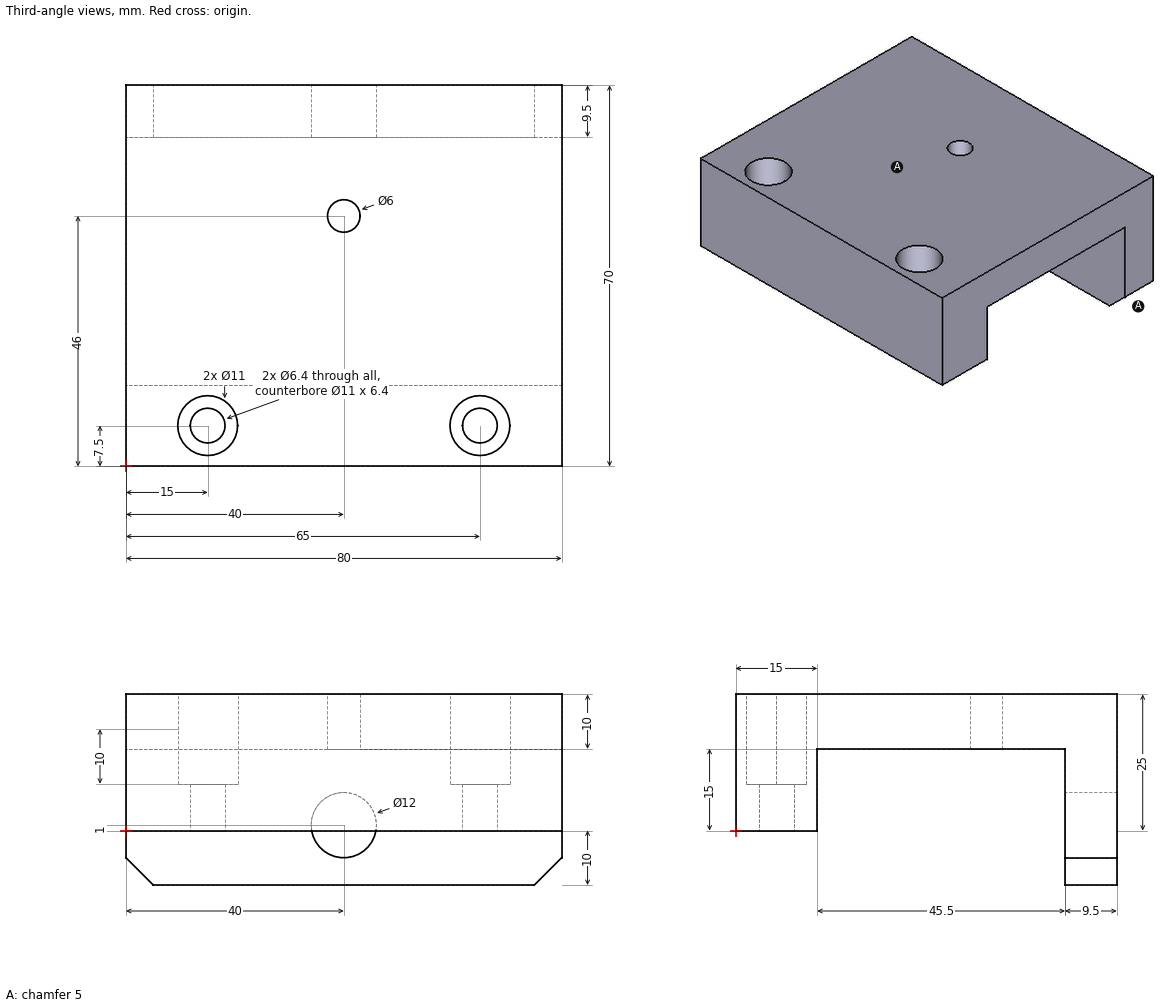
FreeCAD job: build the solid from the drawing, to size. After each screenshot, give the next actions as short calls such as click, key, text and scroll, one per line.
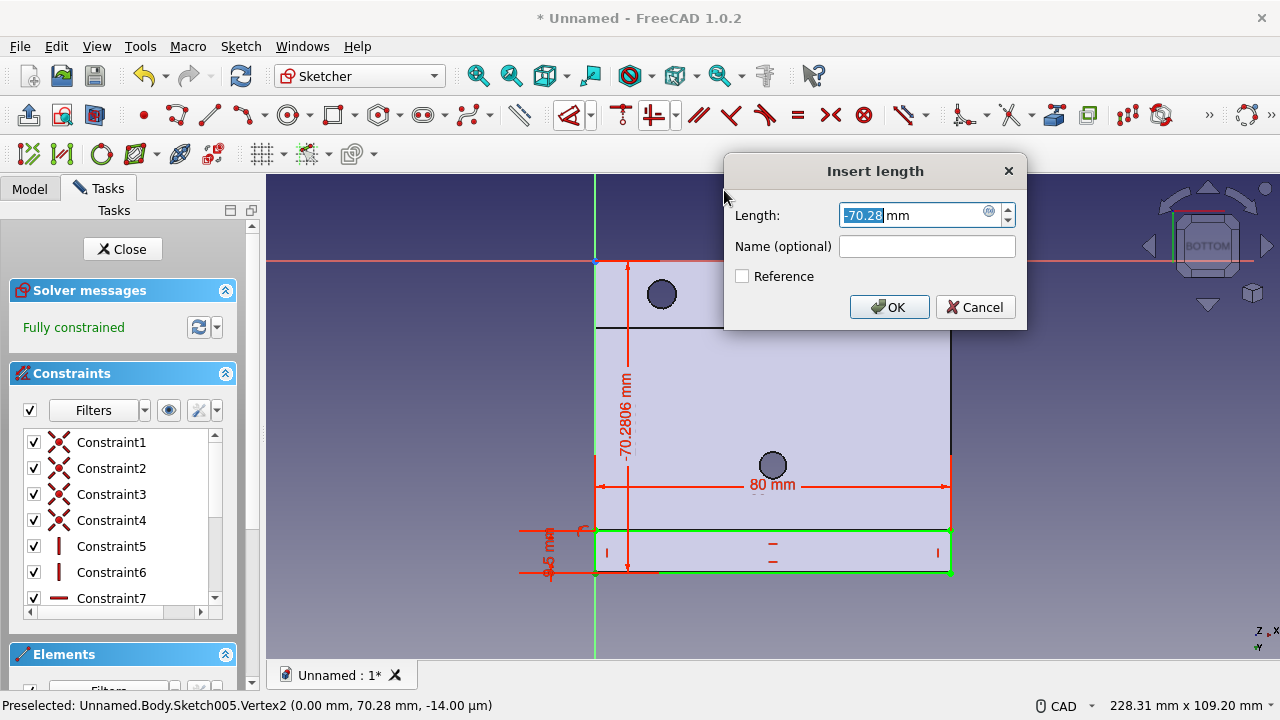
text(-70)
key(Return)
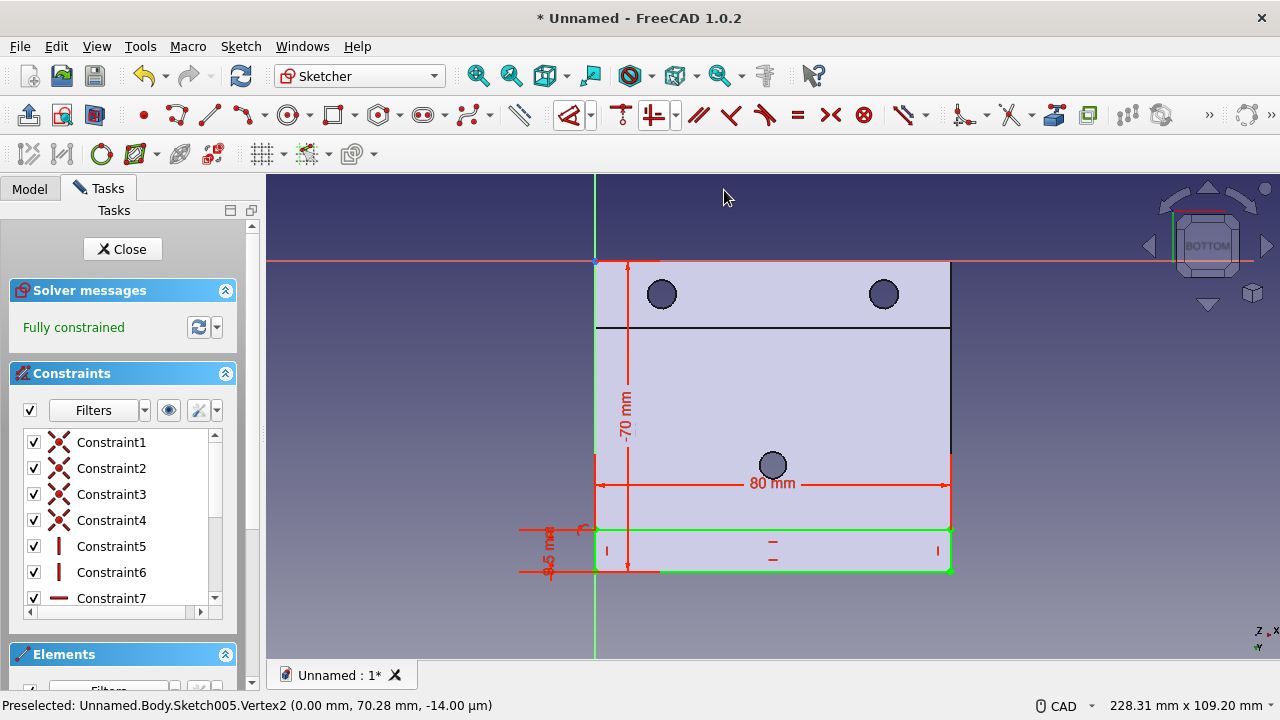
click(123, 249)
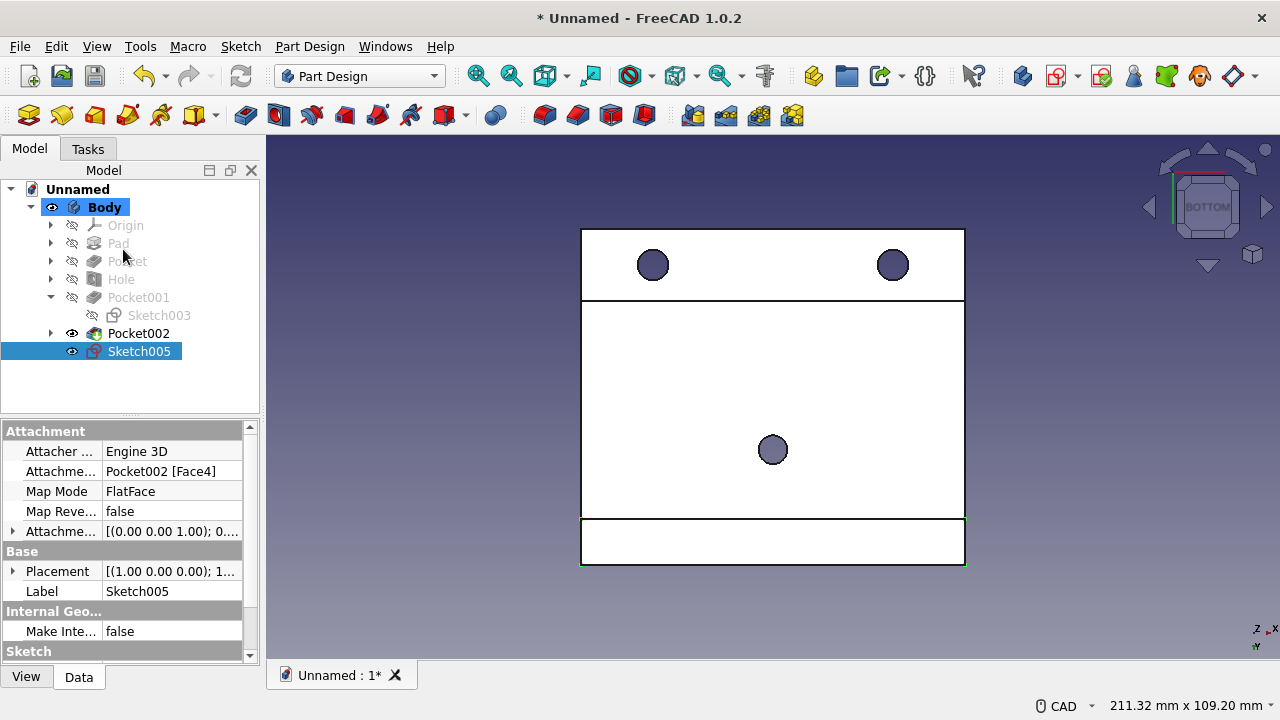
click(29, 116)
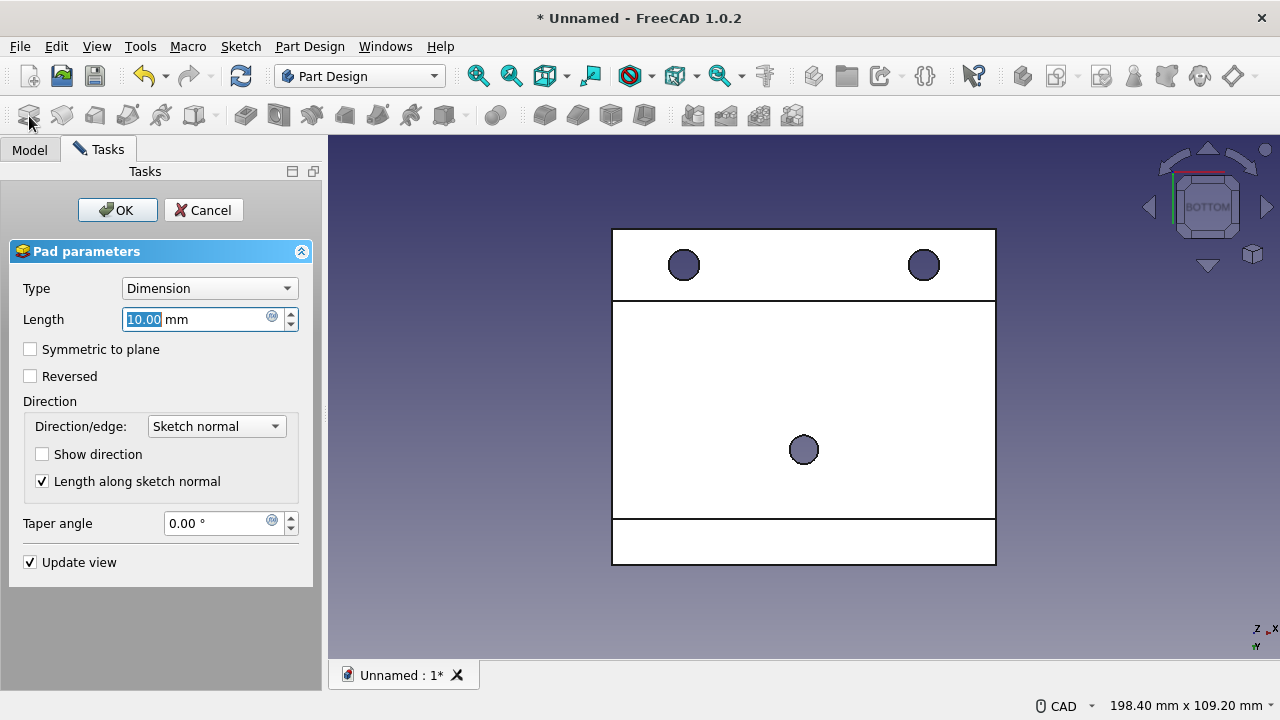
text(10)
key(Tab)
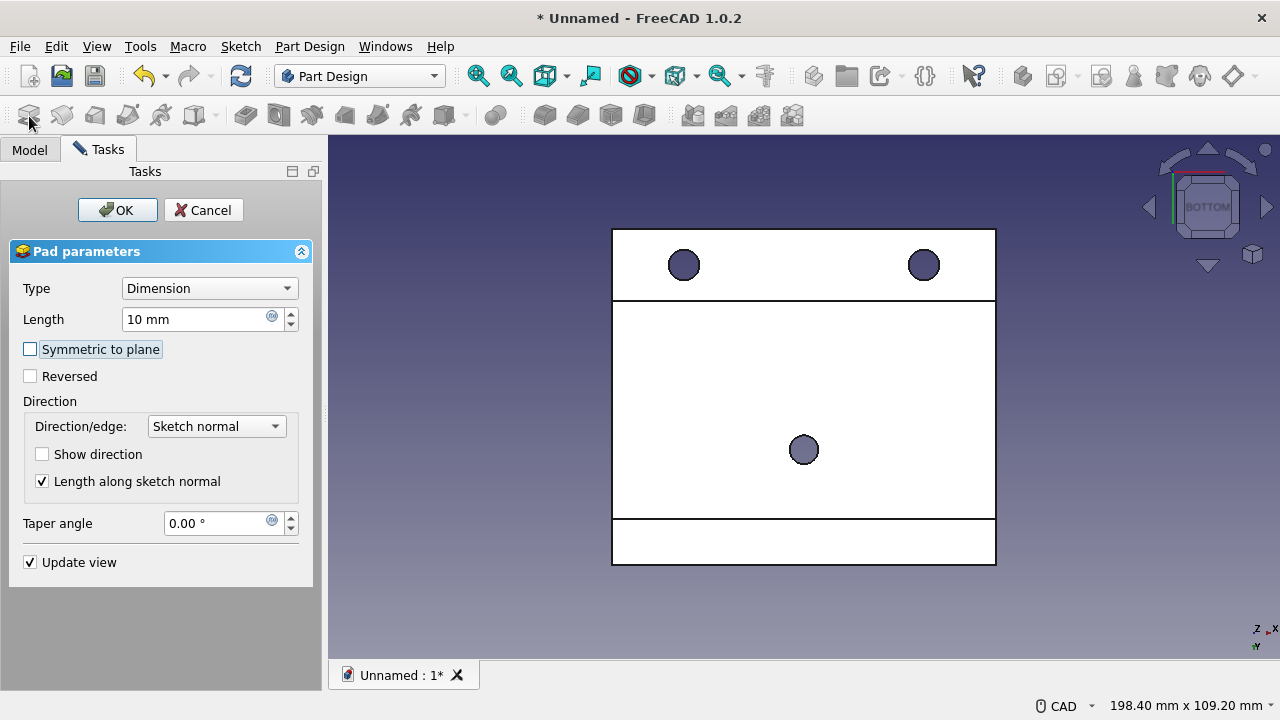
click(118, 210)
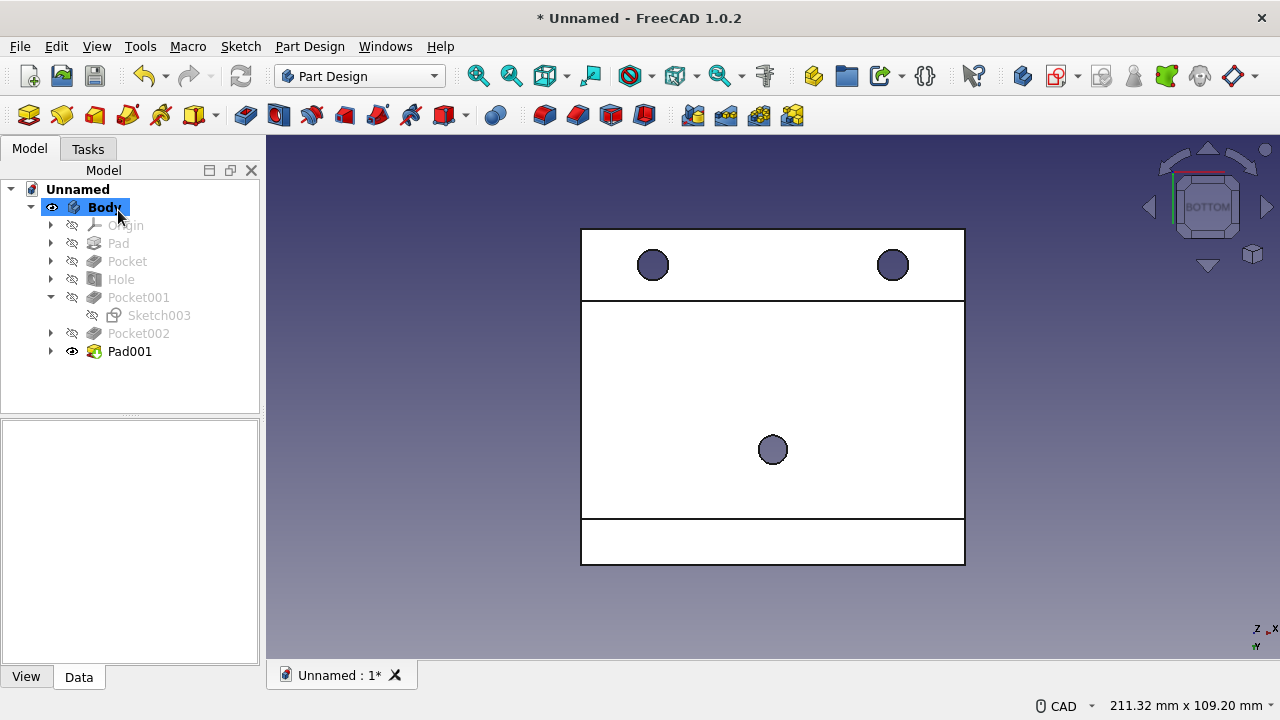
key(4)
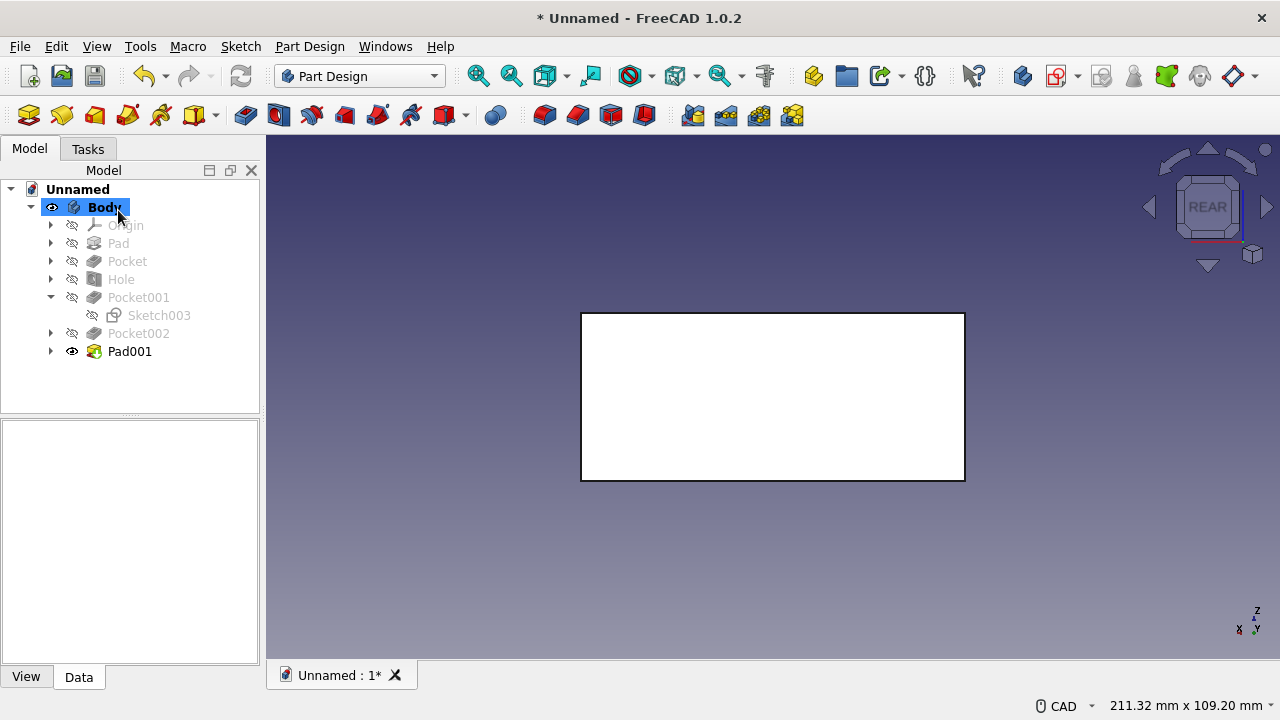
click(479, 76)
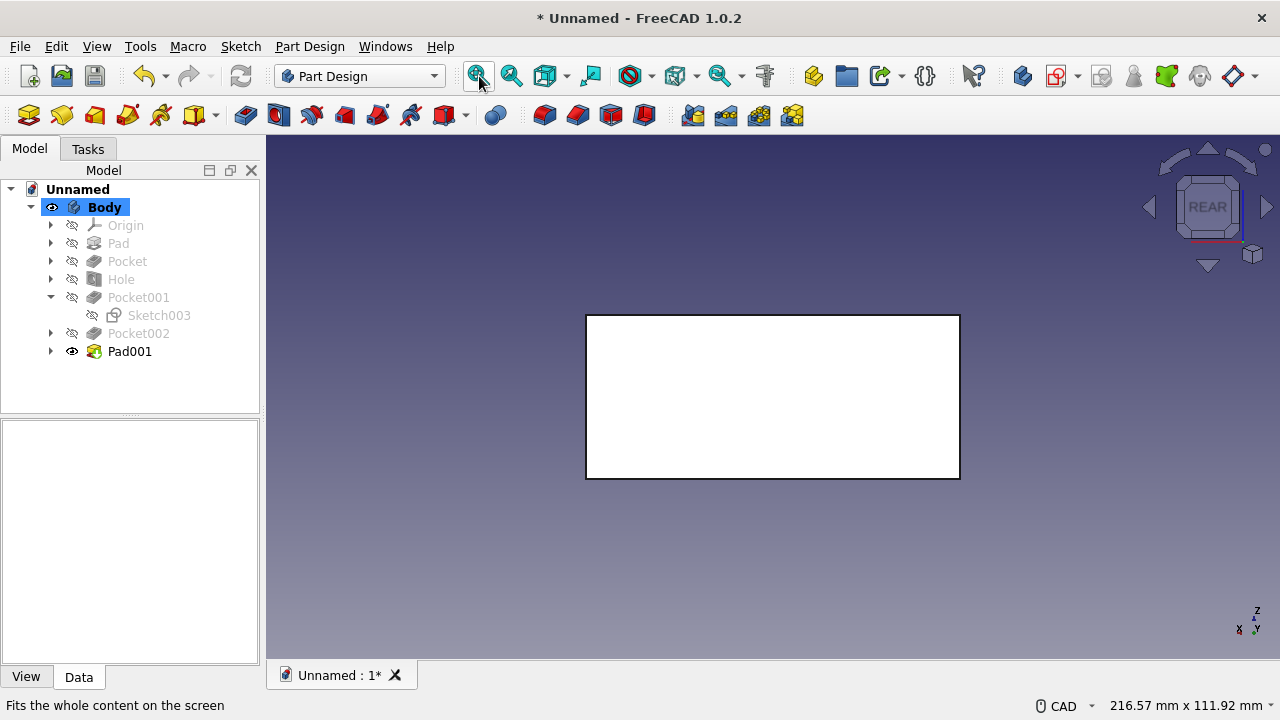
click(719, 396)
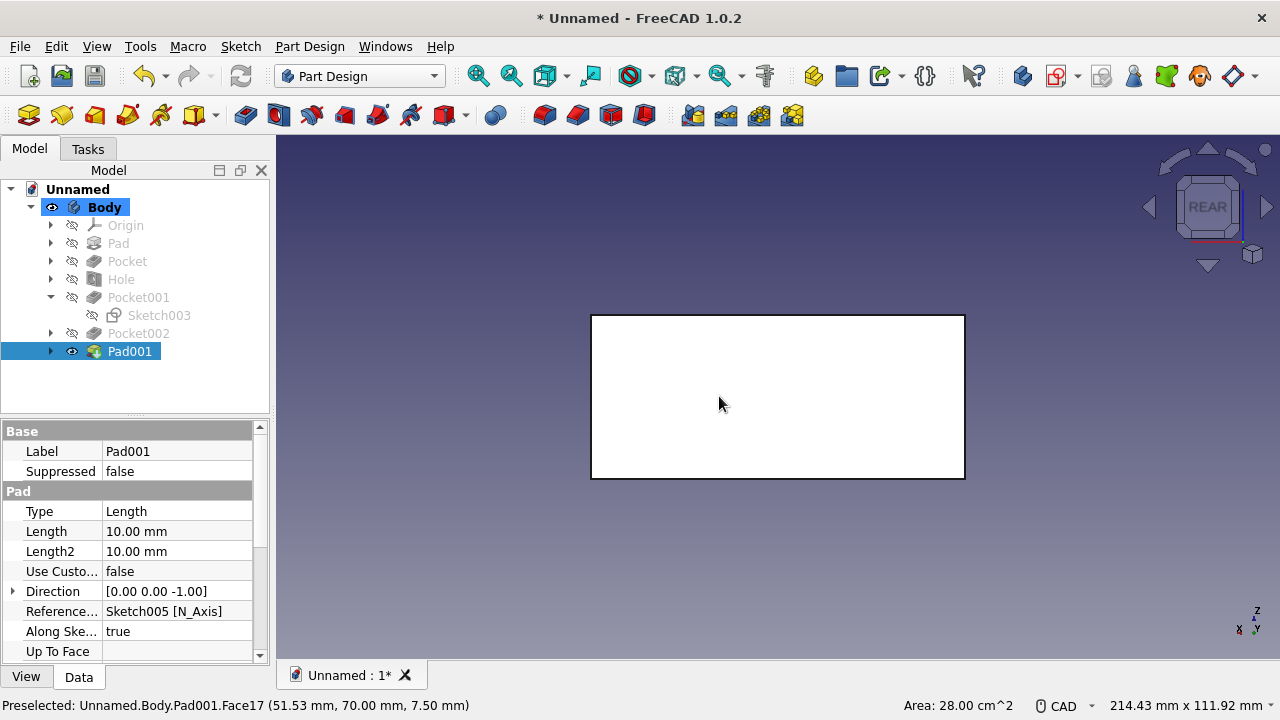
click(1056, 76)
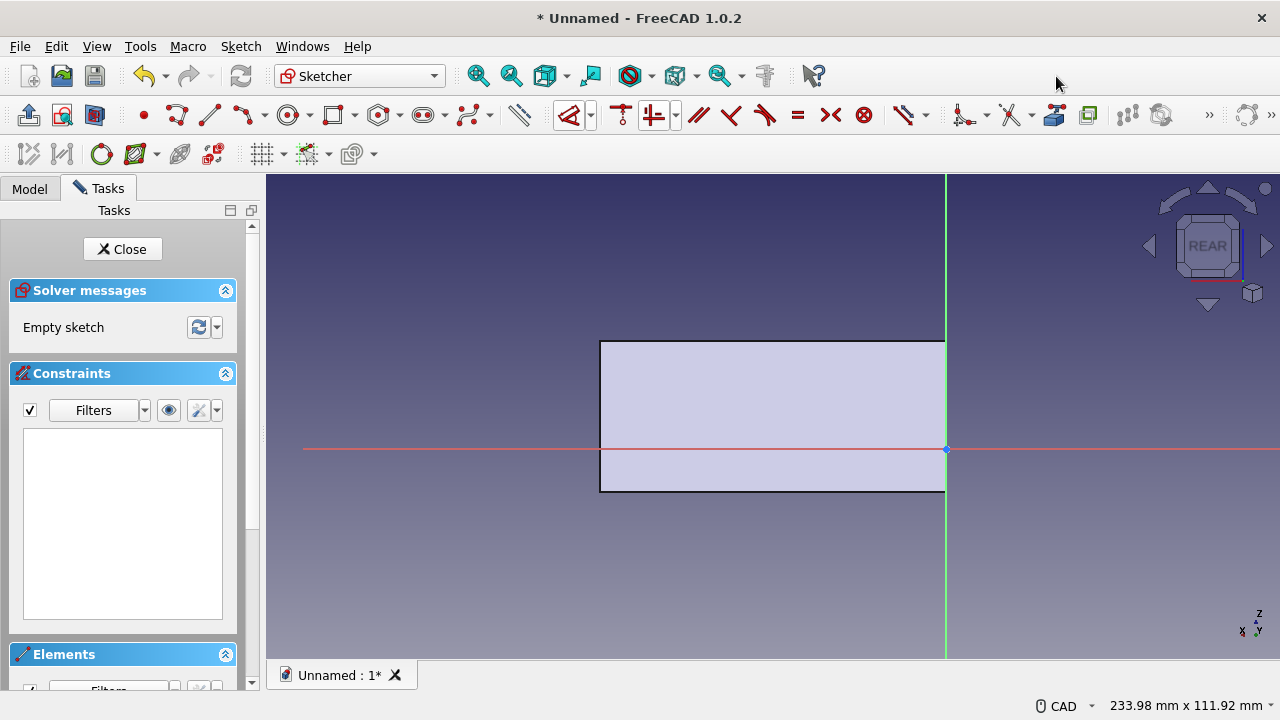
scroll(787, 450, up, 9)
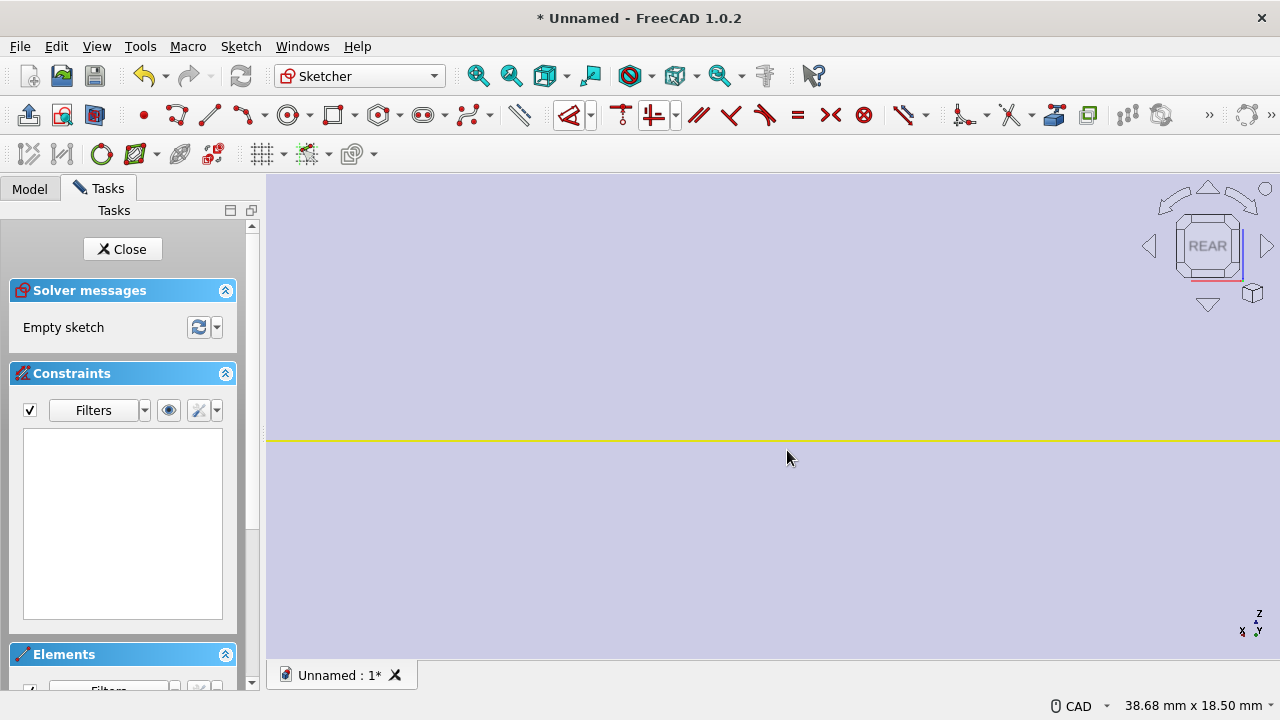
click(288, 116)